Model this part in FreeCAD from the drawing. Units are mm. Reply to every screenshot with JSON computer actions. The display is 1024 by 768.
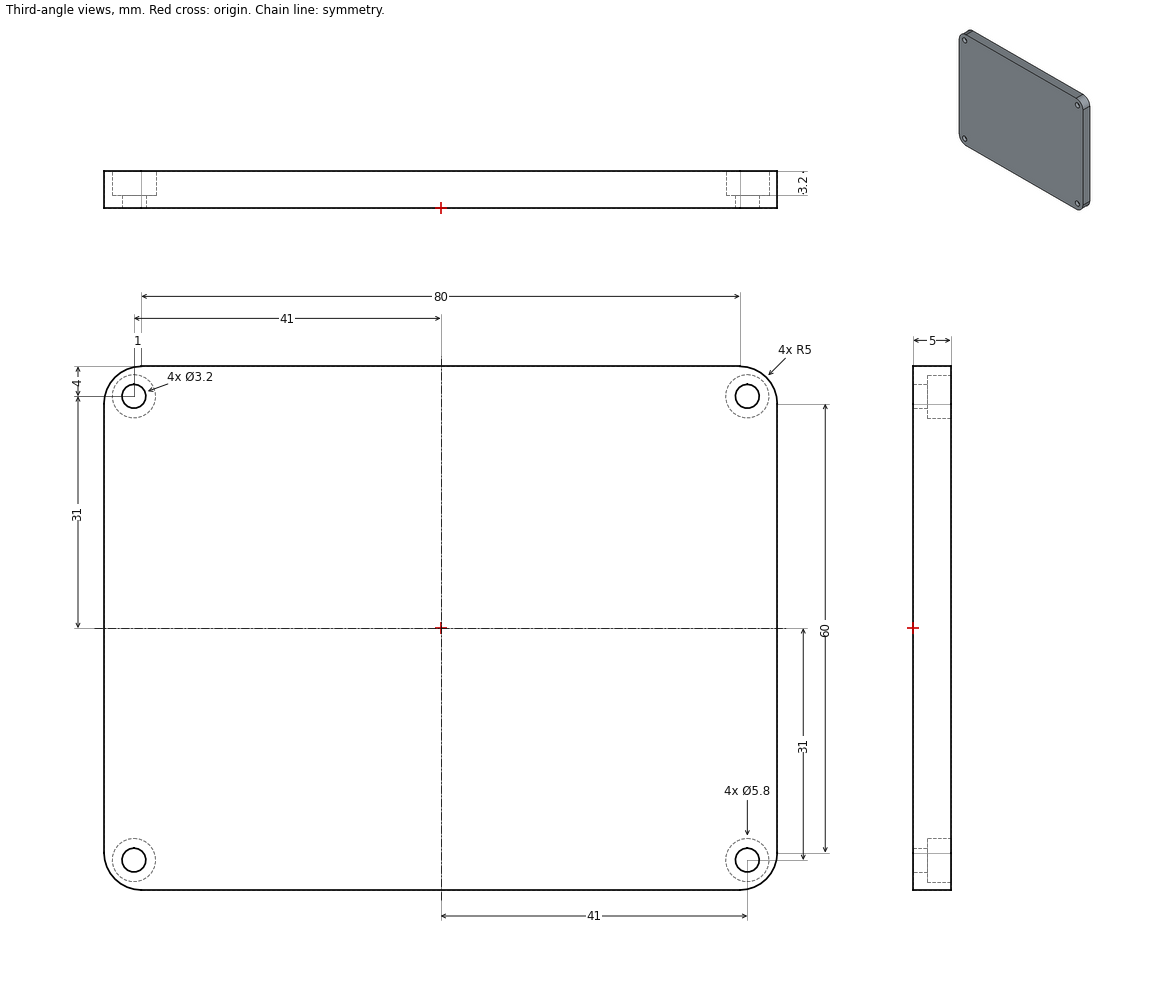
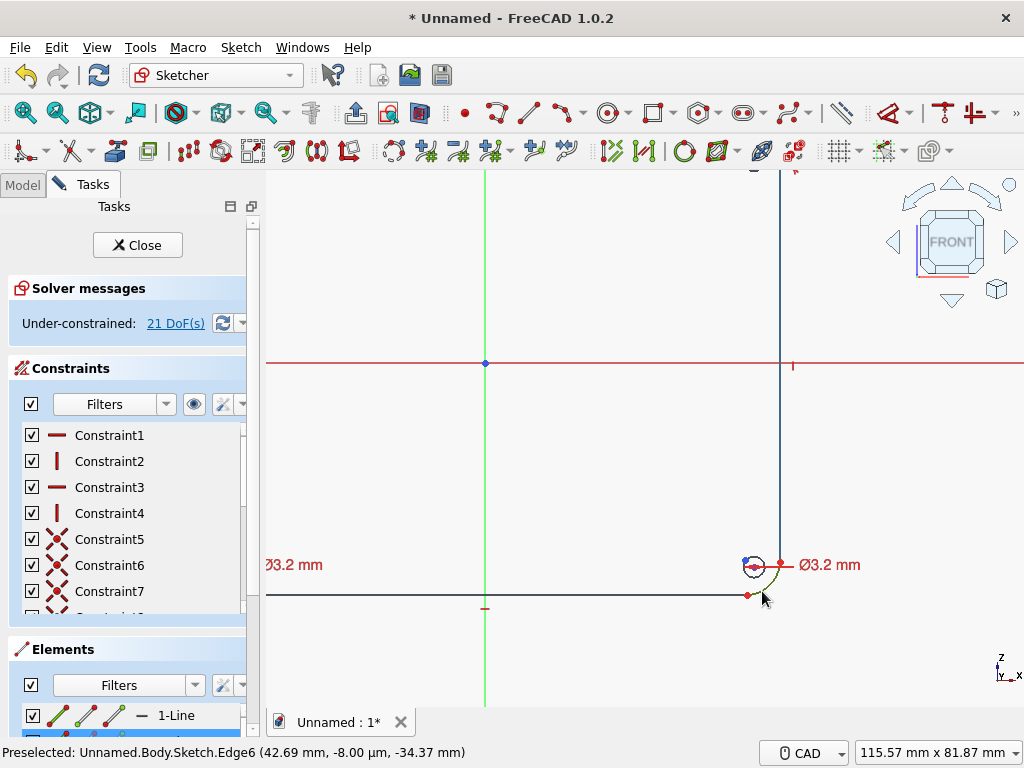
{"action": "key", "text": "t"}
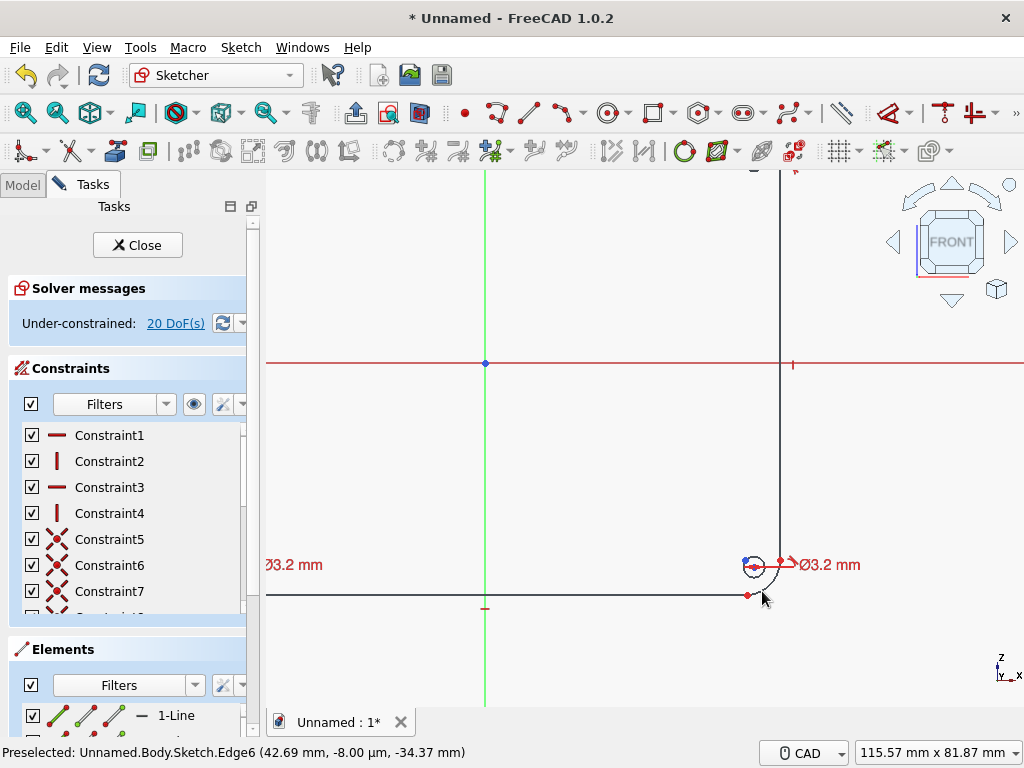
{"action": "left_click", "coordinate": [590, 595]}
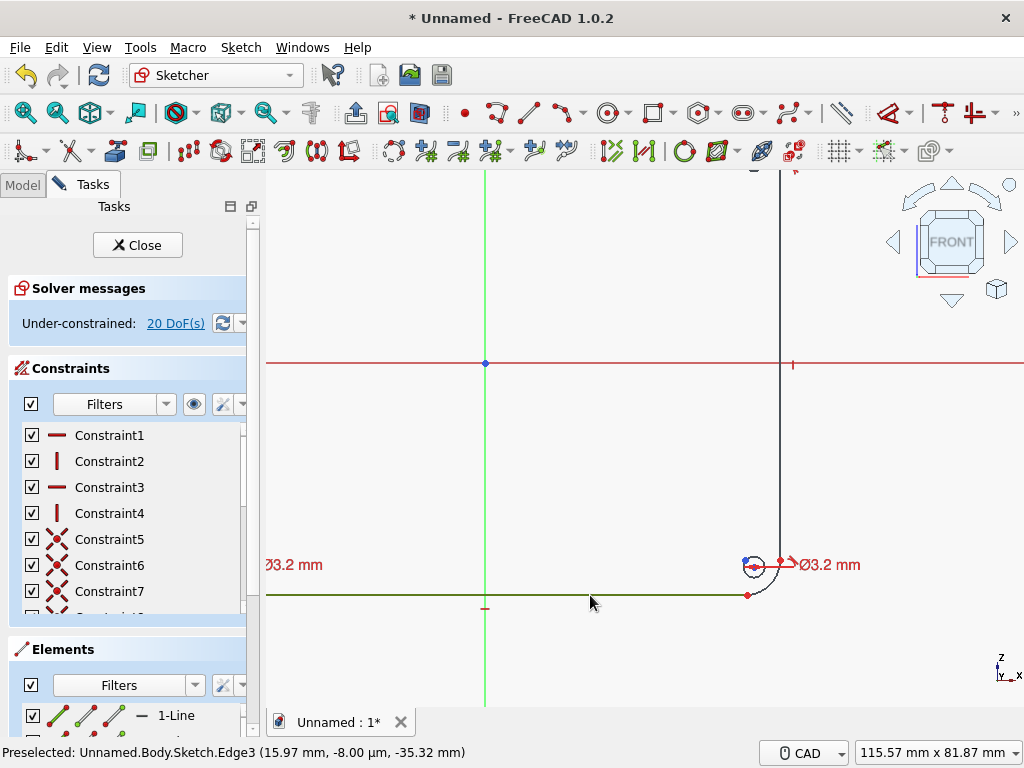
{"action": "left_click", "coordinate": [762, 591]}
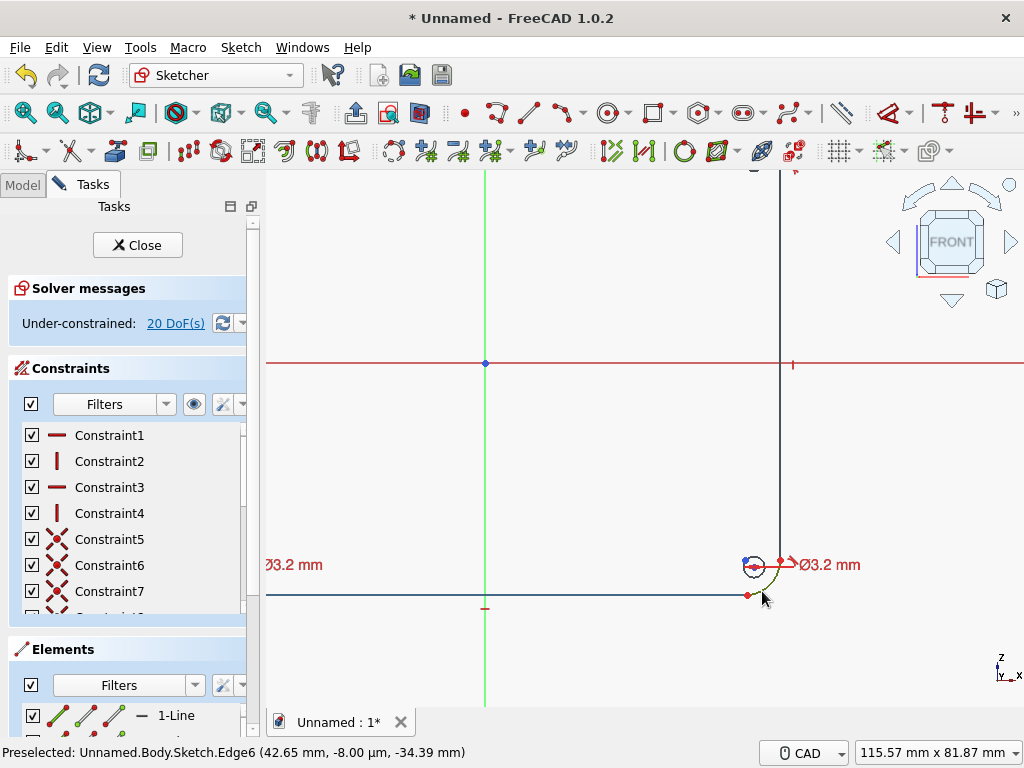
{"action": "key", "text": "t"}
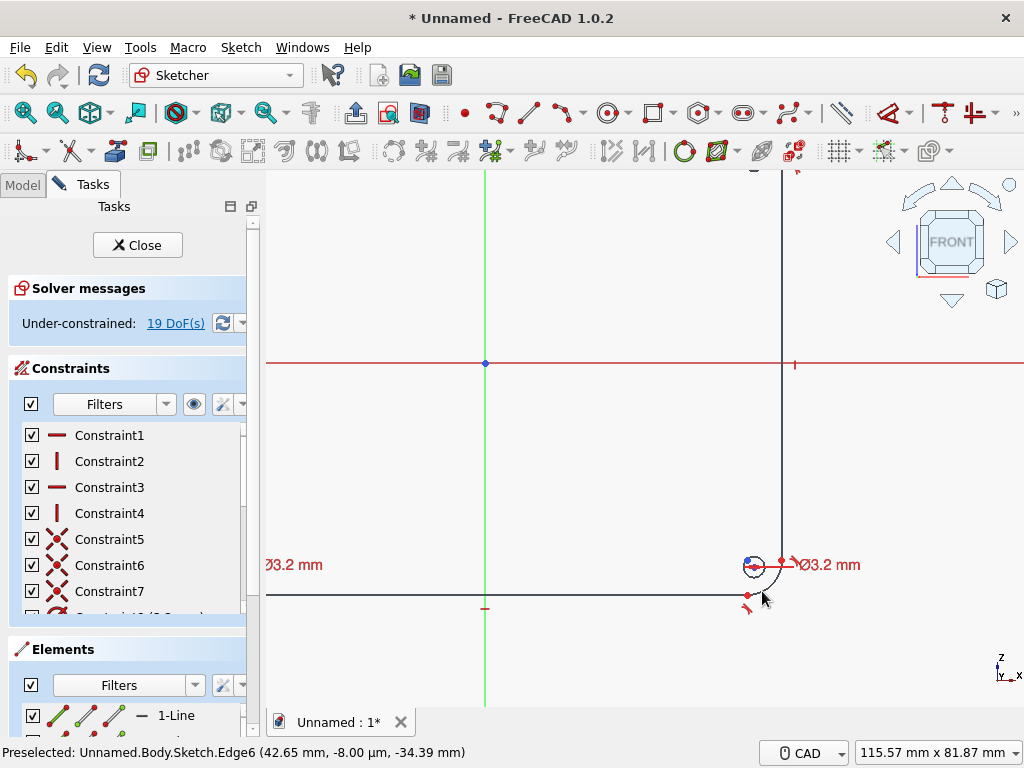
{"action": "left_click", "coordinate": [590, 595]}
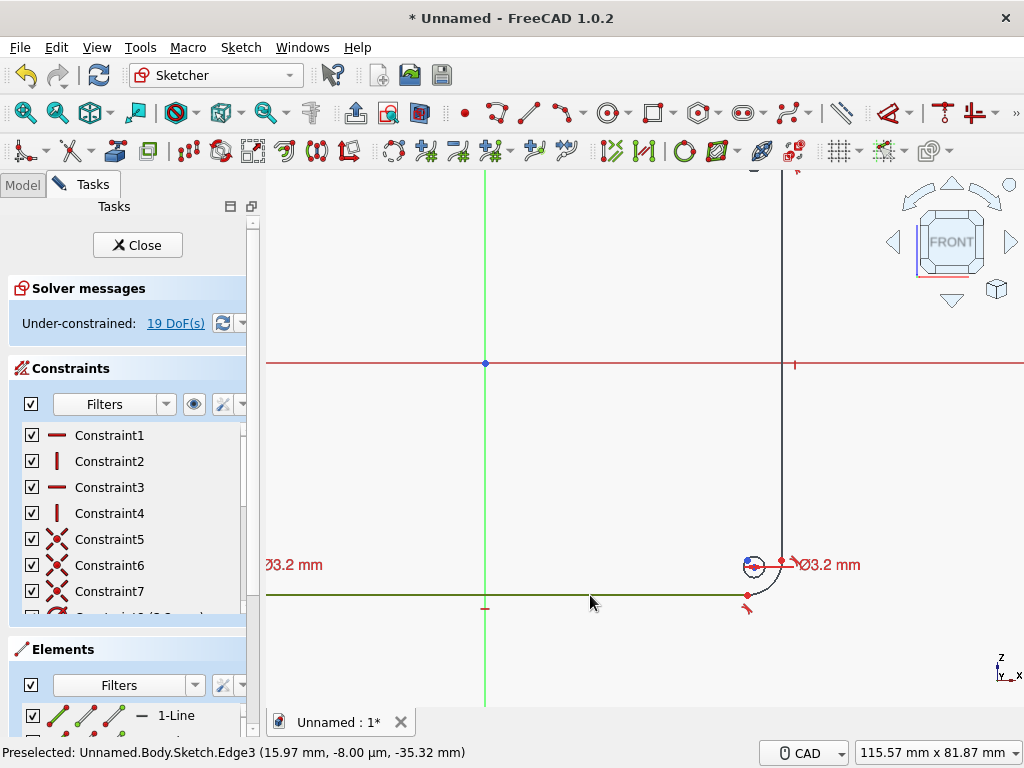
{"action": "scroll", "coordinate": [762, 591], "scroll_direction": "down", "scroll_amount": 2}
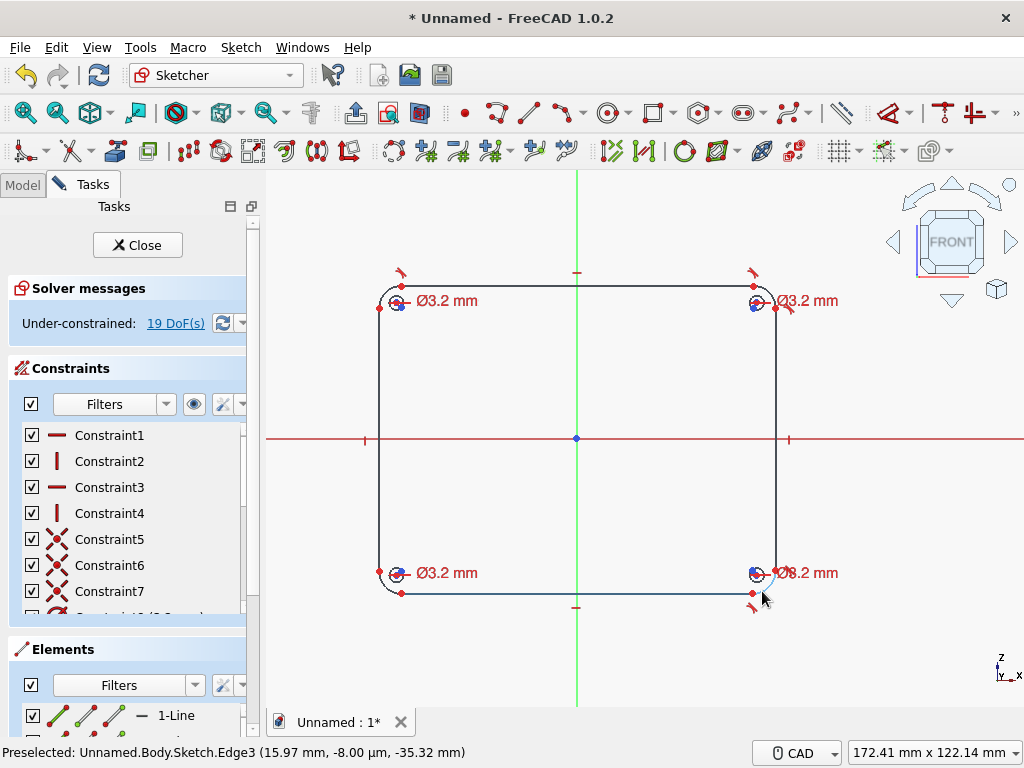
{"action": "scroll", "coordinate": [382, 582], "scroll_direction": "up", "scroll_amount": 3}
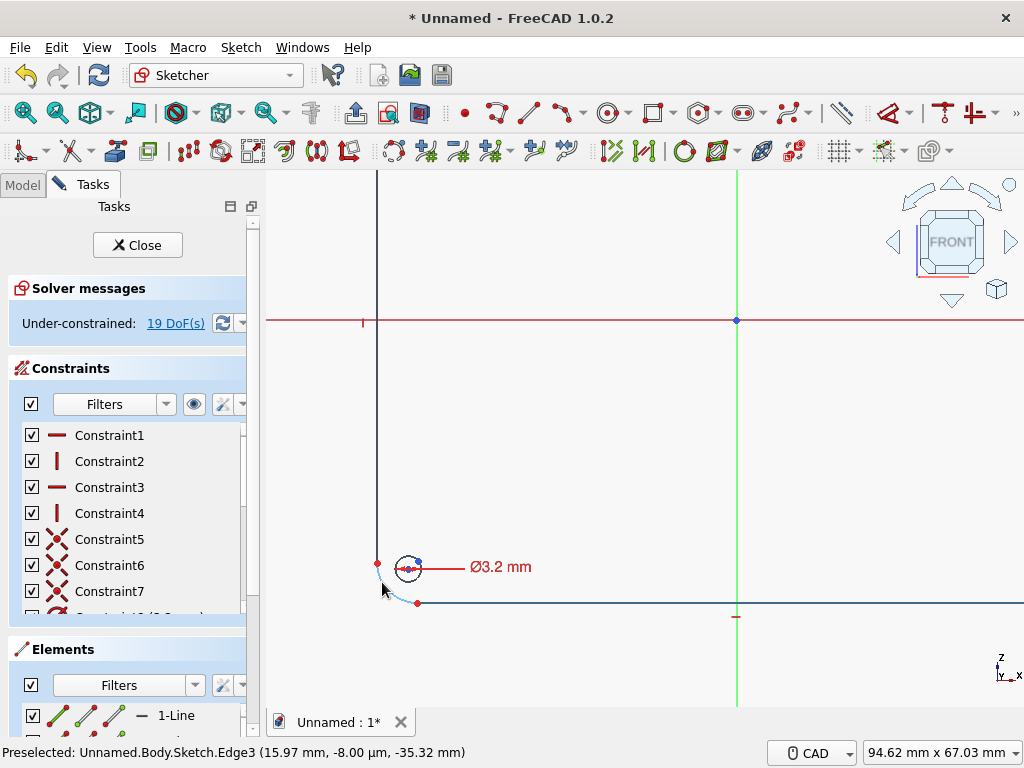
{"action": "left_click", "coordinate": [382, 581]}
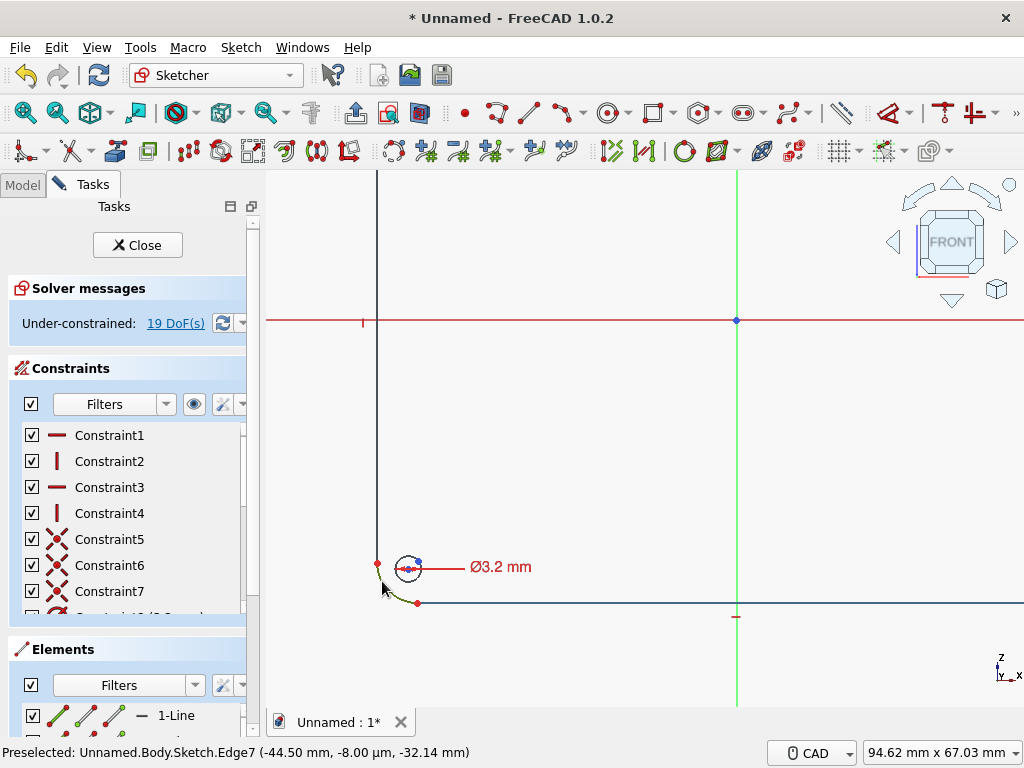
{"action": "key", "text": "t"}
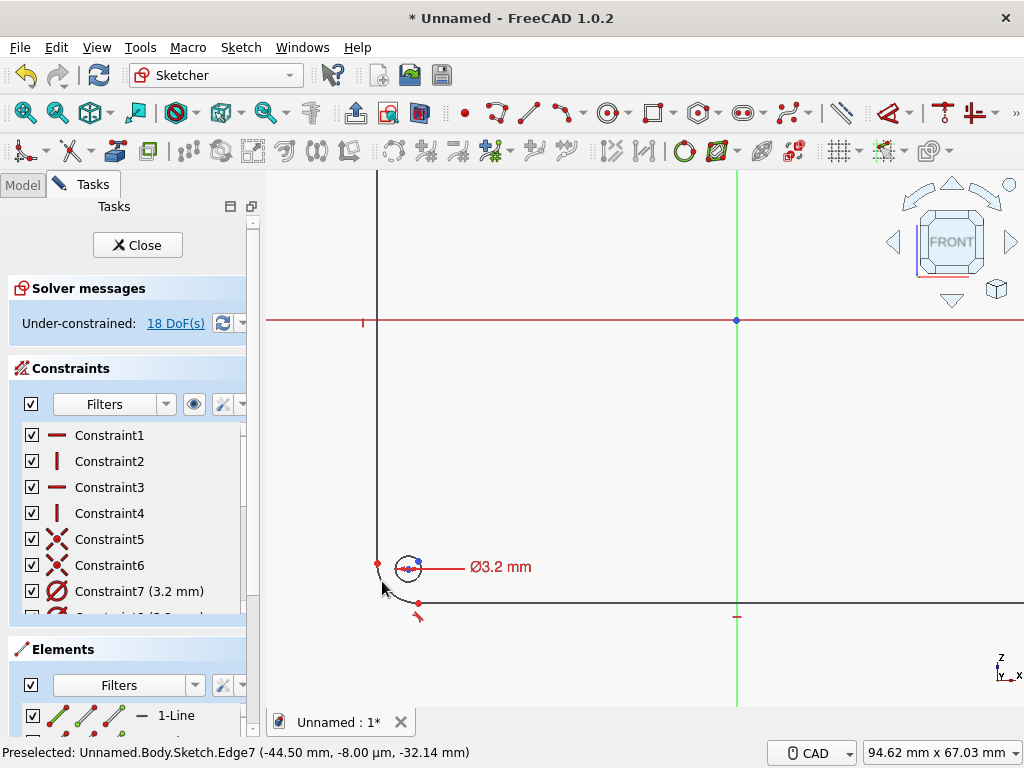
{"action": "left_click", "coordinate": [377, 419]}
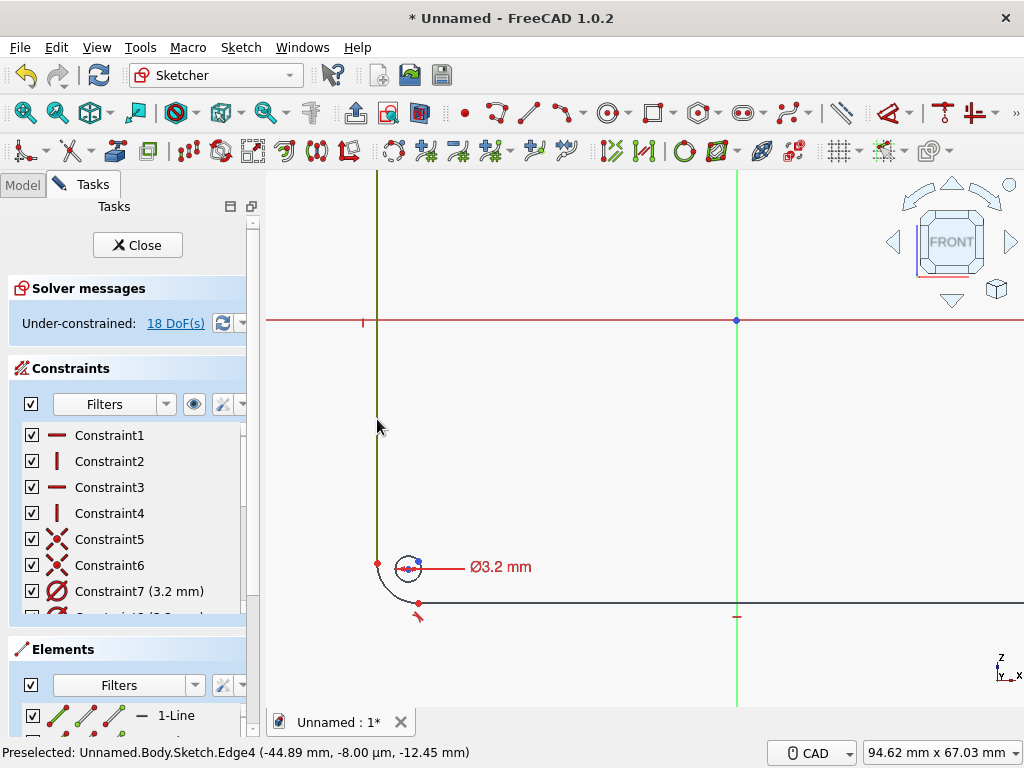
{"action": "left_click", "coordinate": [382, 581]}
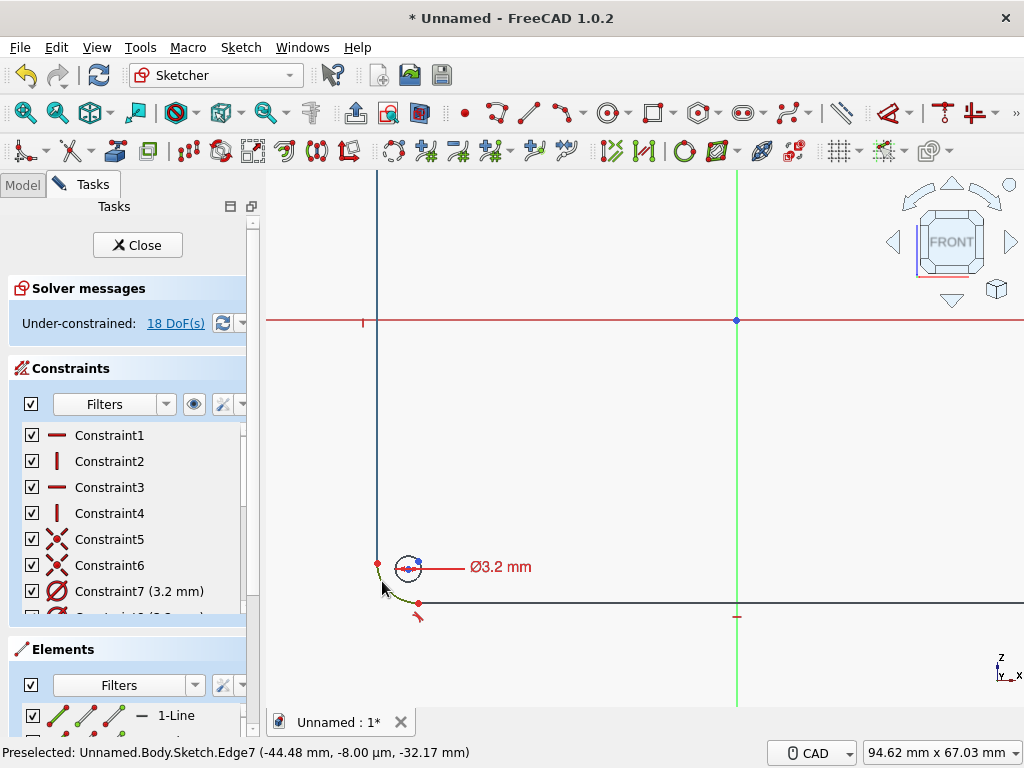
{"action": "key", "text": "t"}